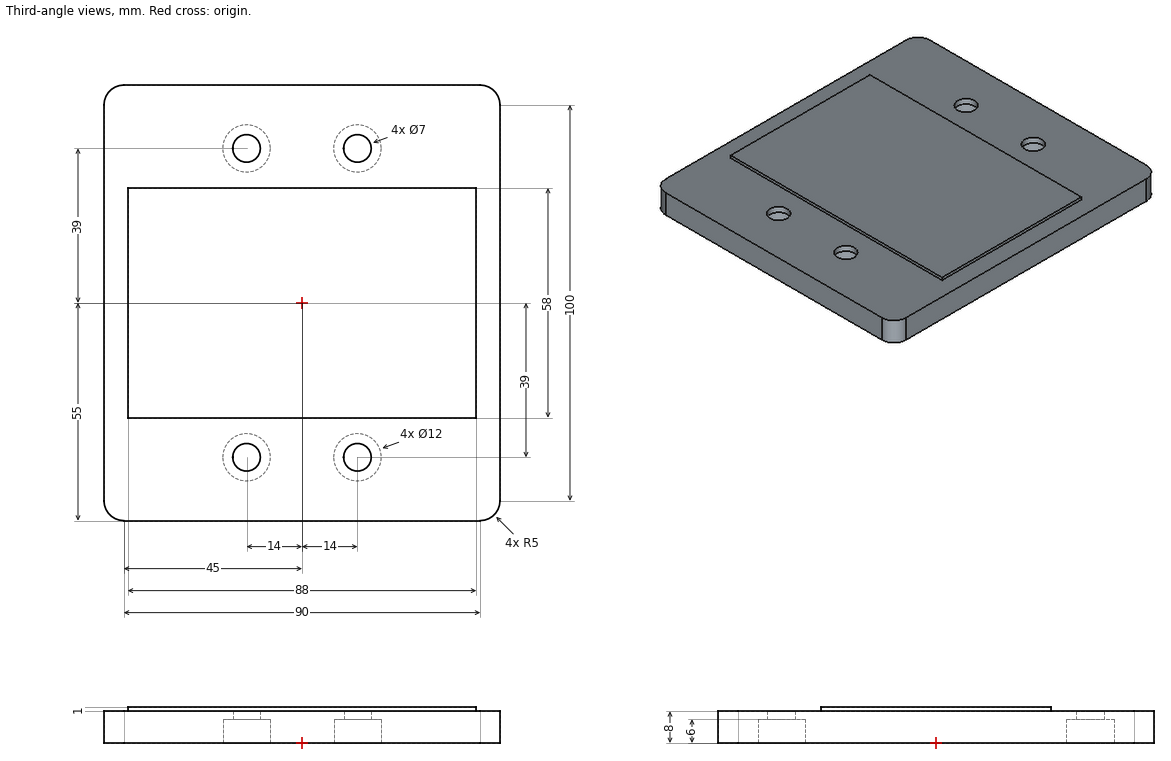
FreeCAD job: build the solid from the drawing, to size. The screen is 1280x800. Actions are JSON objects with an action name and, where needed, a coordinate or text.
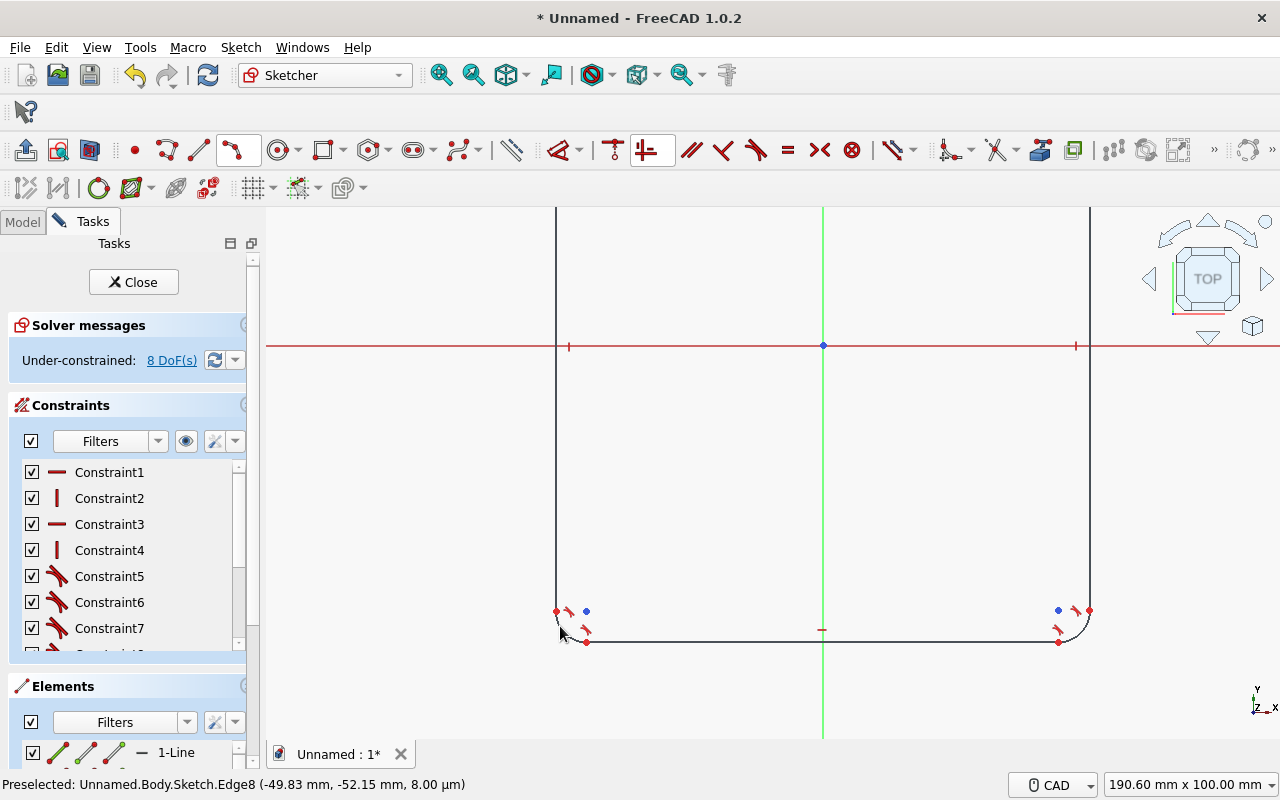
{"action": "left_click", "coordinate": [1073, 639]}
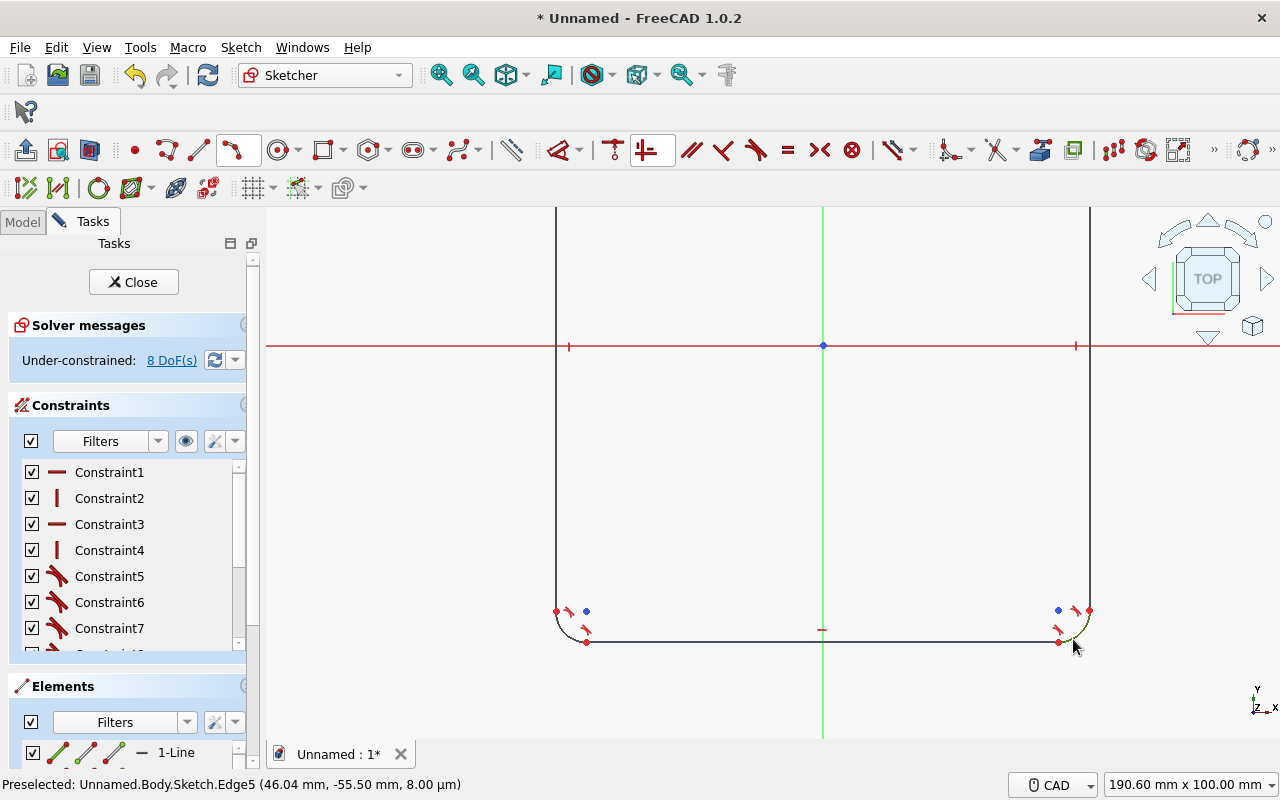
{"action": "scroll", "coordinate": [560, 628], "scroll_direction": "down", "scroll_amount": 3}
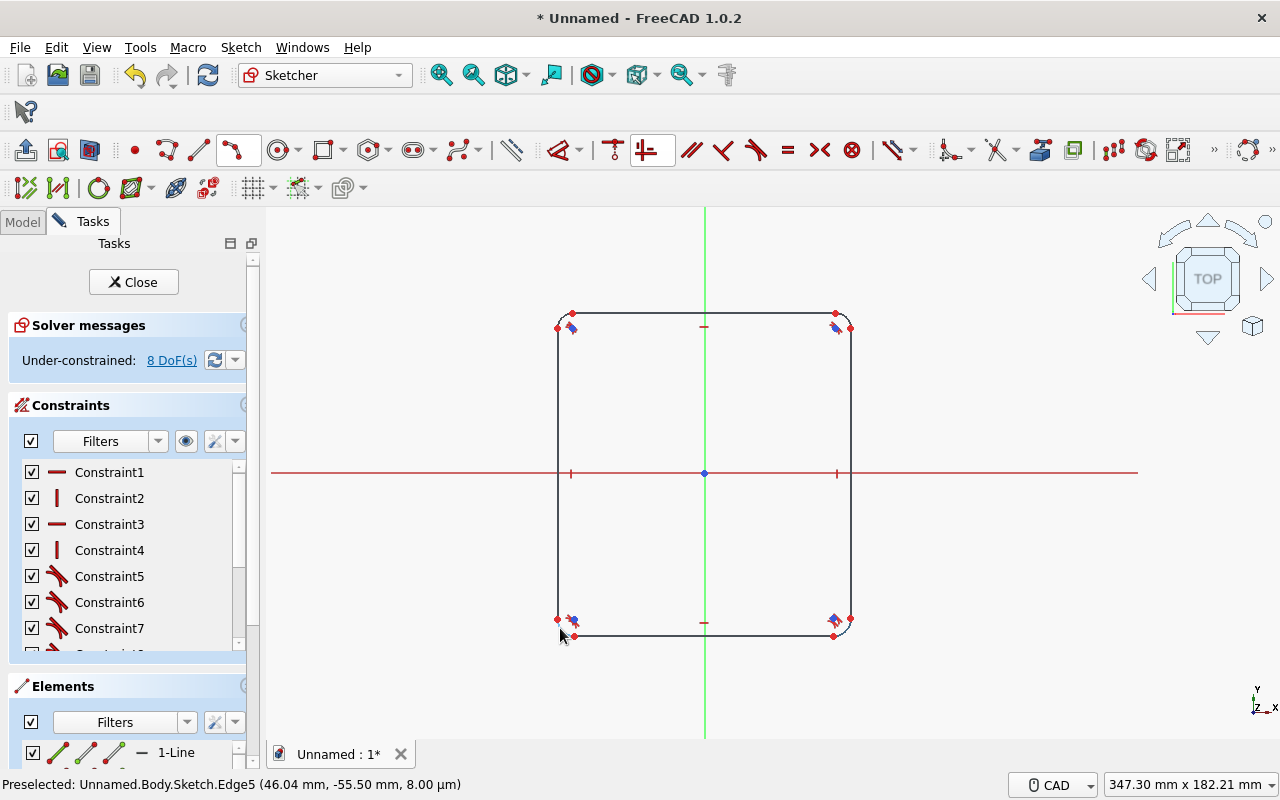
{"action": "scroll", "coordinate": [849, 321], "scroll_direction": "up", "scroll_amount": 4}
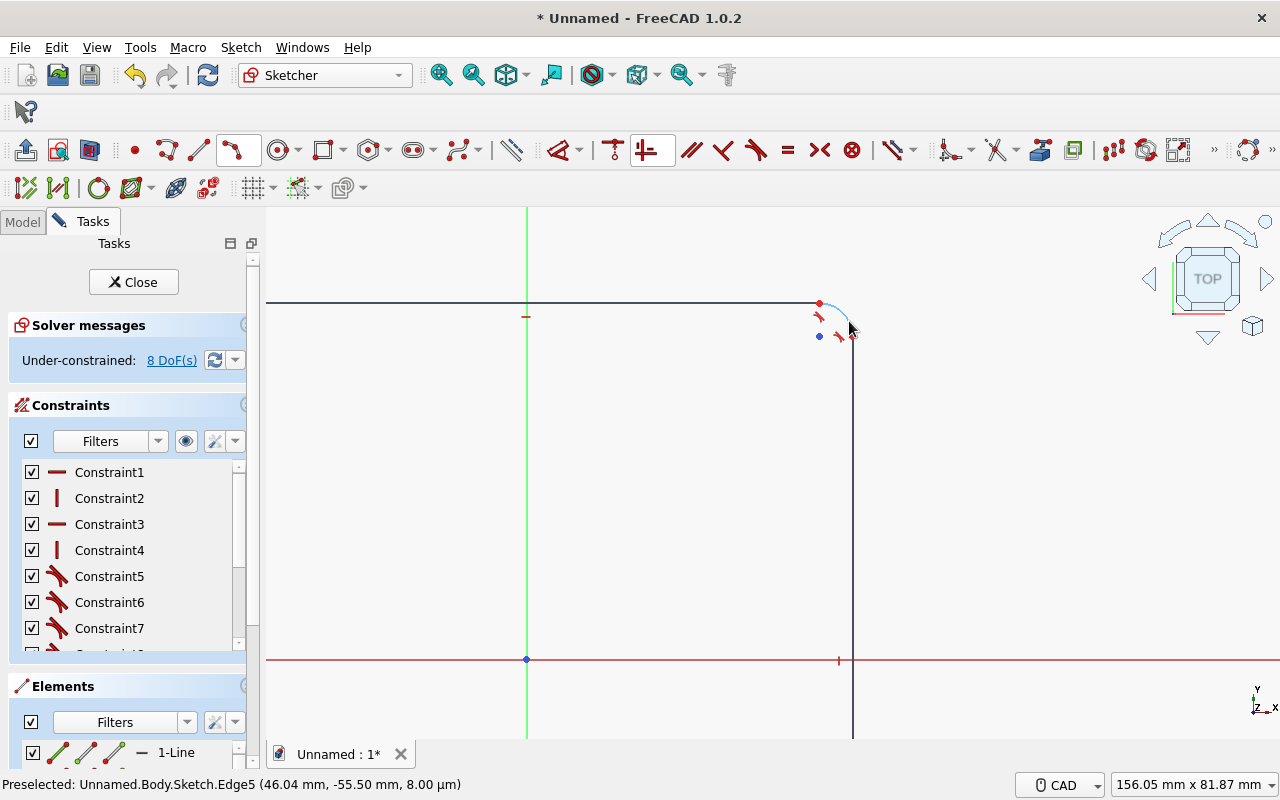
{"action": "left_click", "coordinate": [849, 321]}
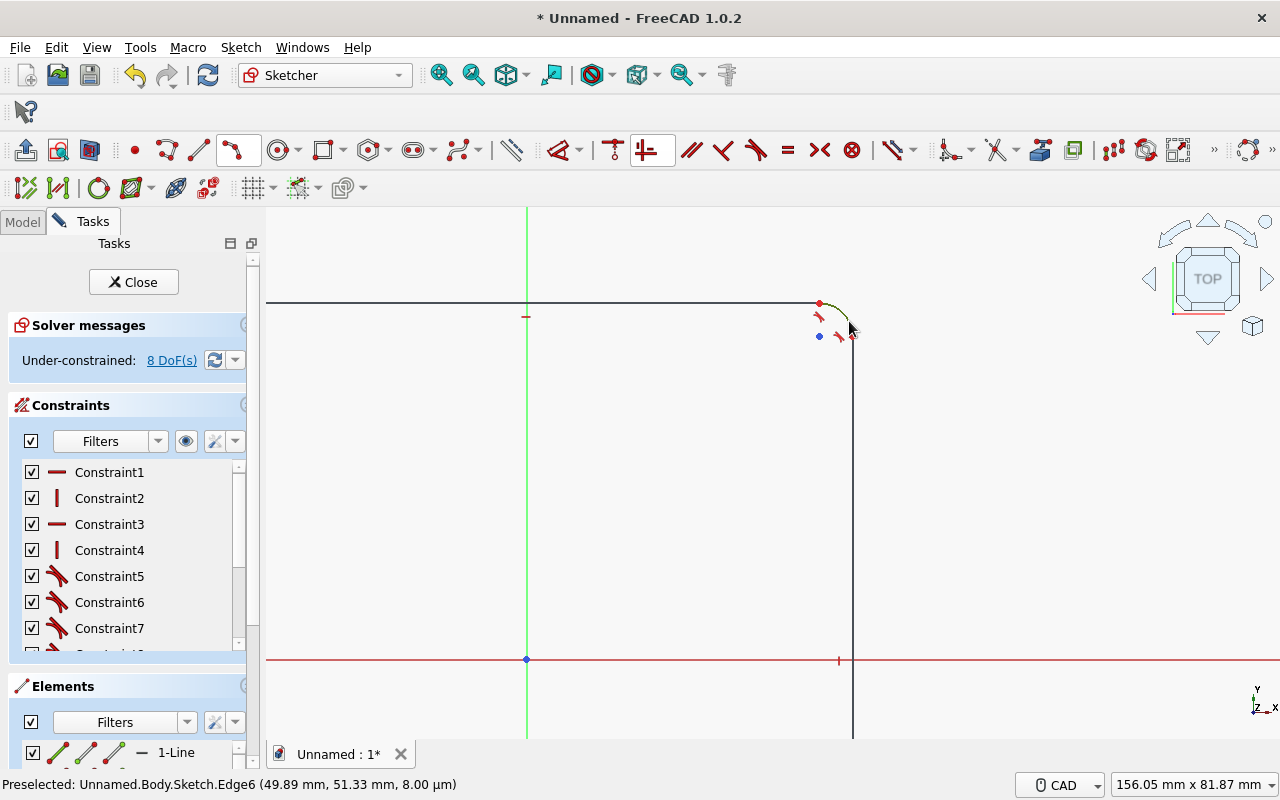
{"action": "scroll", "coordinate": [849, 321], "scroll_direction": "down", "scroll_amount": 4}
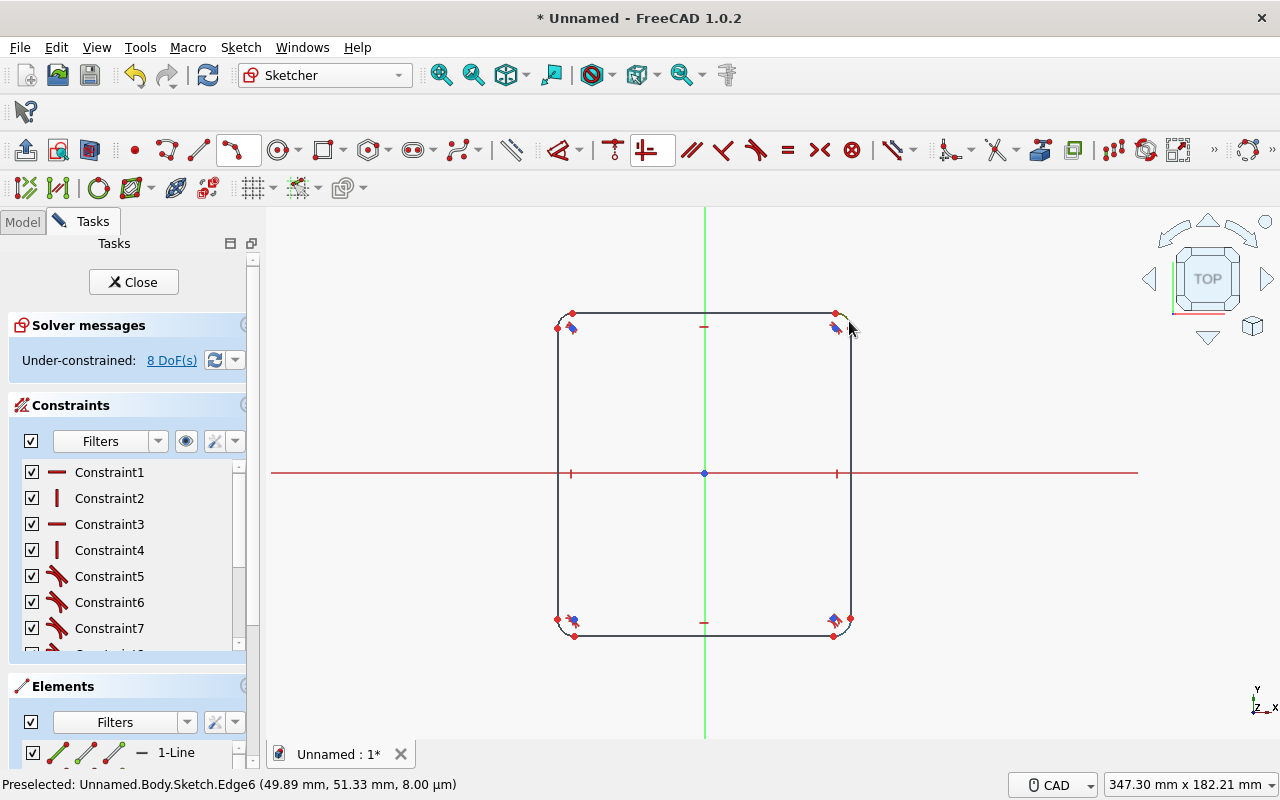
{"action": "scroll", "coordinate": [566, 315], "scroll_direction": "up", "scroll_amount": 4}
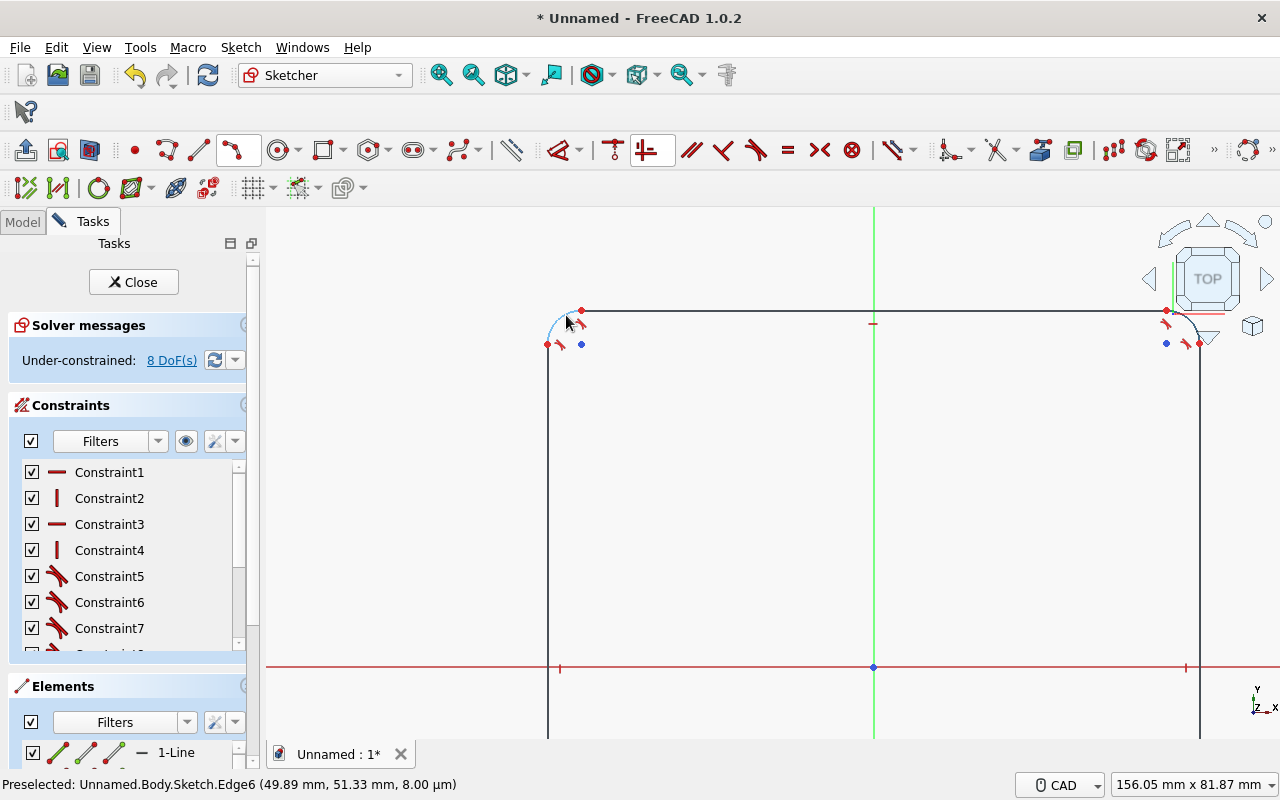
{"action": "left_click", "coordinate": [566, 314]}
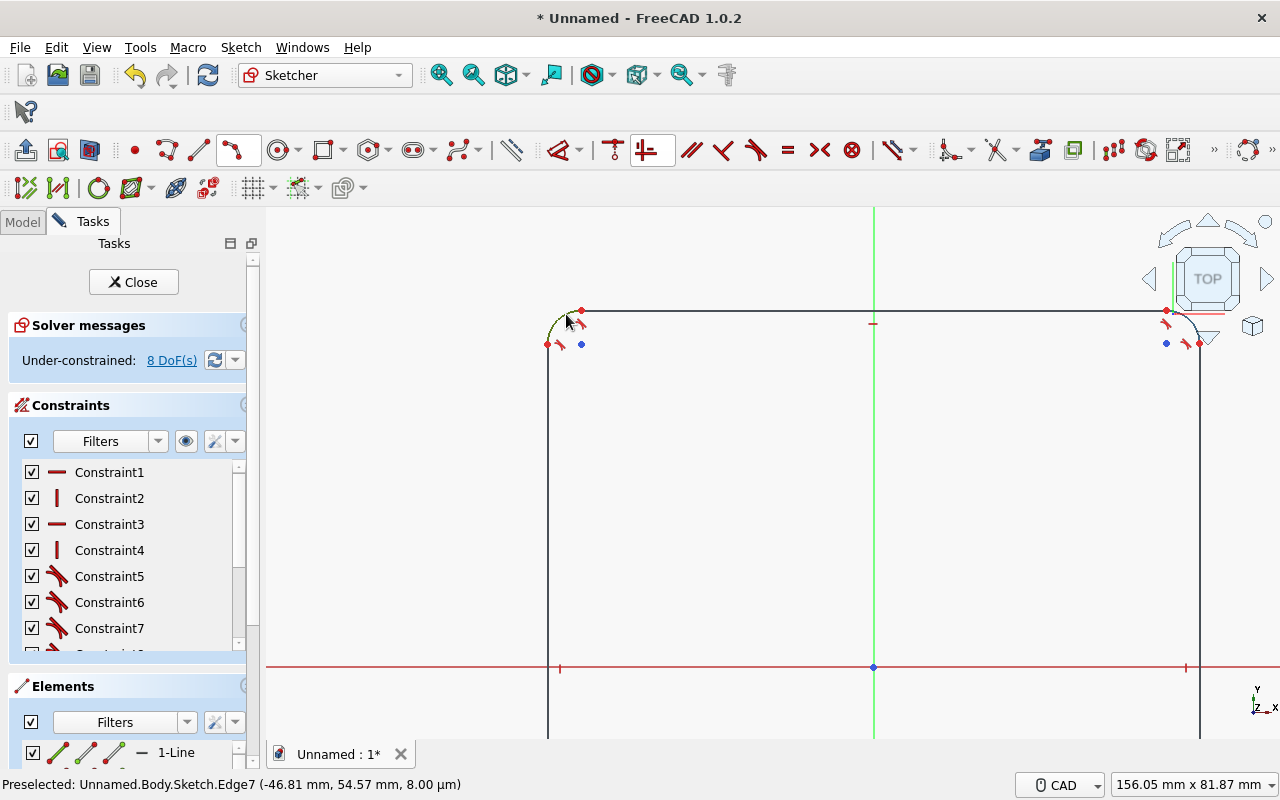
{"action": "scroll", "coordinate": [566, 315], "scroll_direction": "down", "scroll_amount": 4}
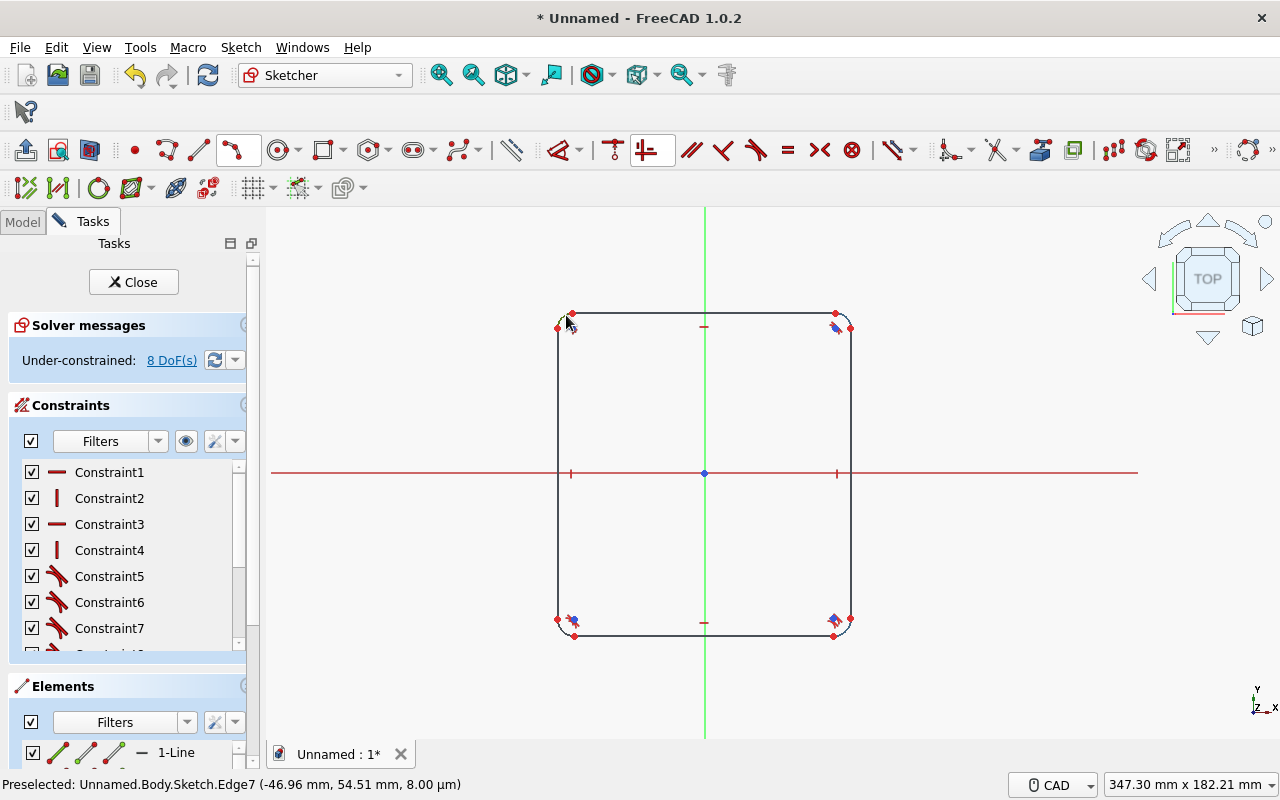
{"action": "scroll", "coordinate": [560, 627], "scroll_direction": "up", "scroll_amount": 3}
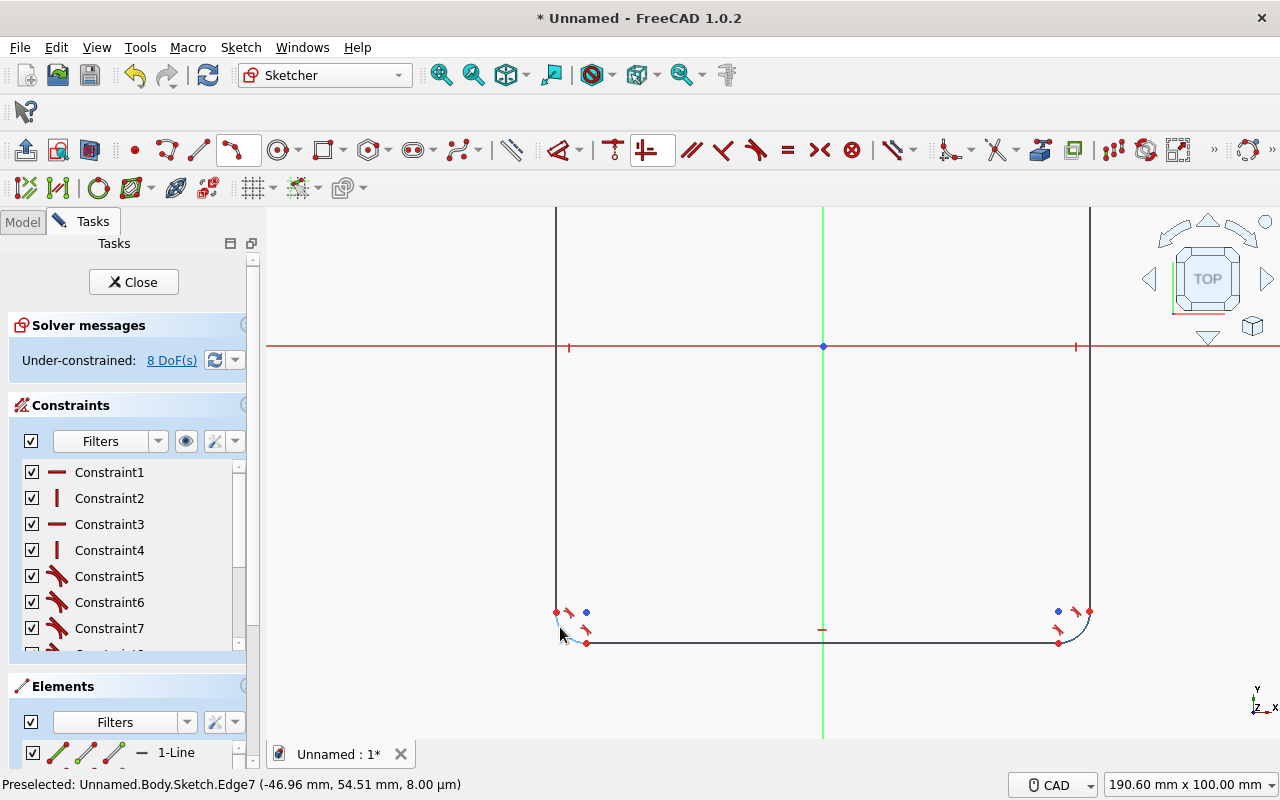
{"action": "left_click", "coordinate": [559, 627]}